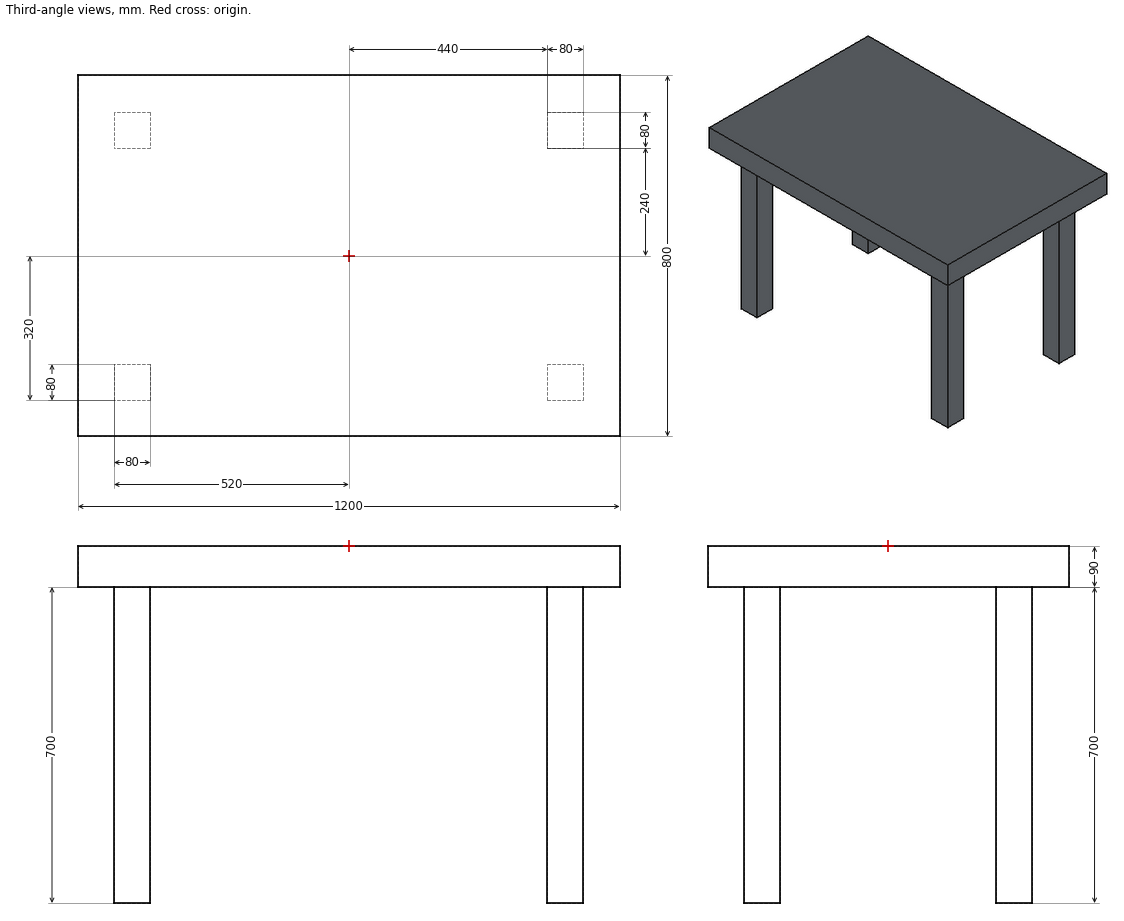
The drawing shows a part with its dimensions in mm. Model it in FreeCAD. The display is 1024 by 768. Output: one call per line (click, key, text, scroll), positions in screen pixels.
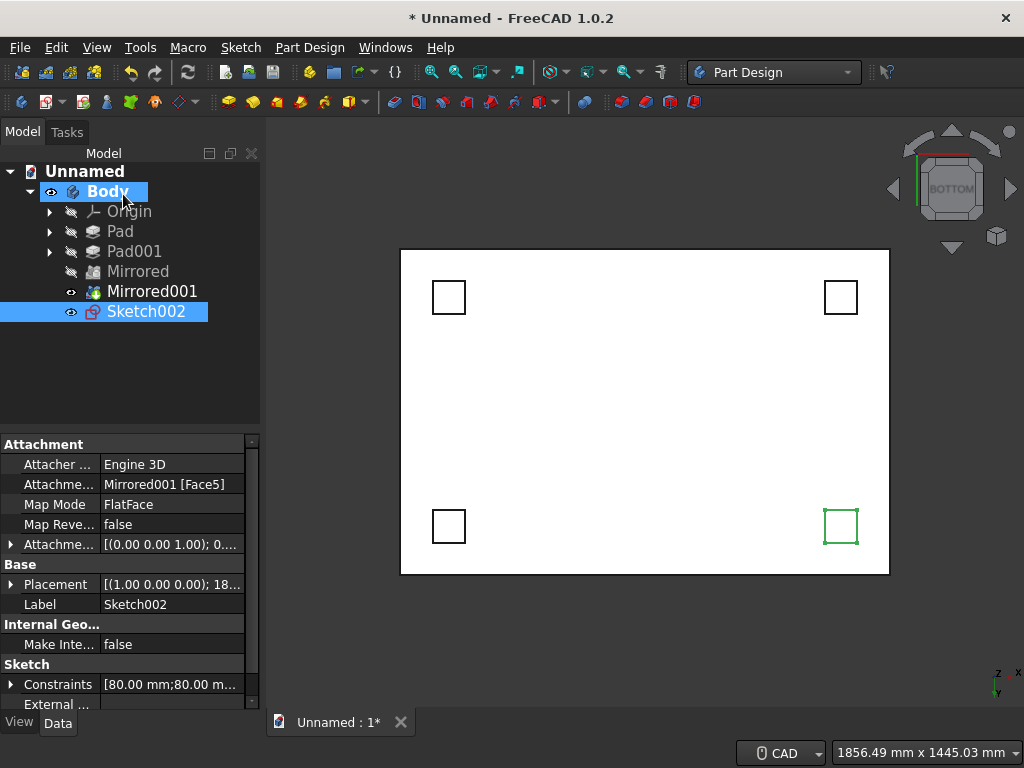
click(230, 102)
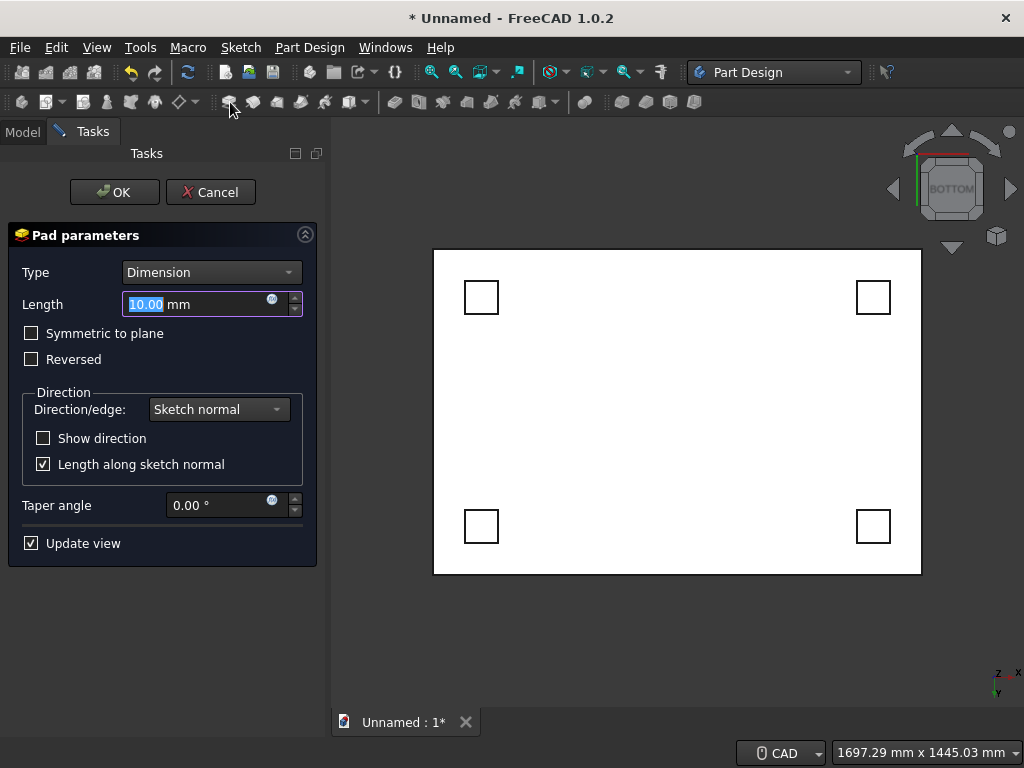
text(700)
key(Tab)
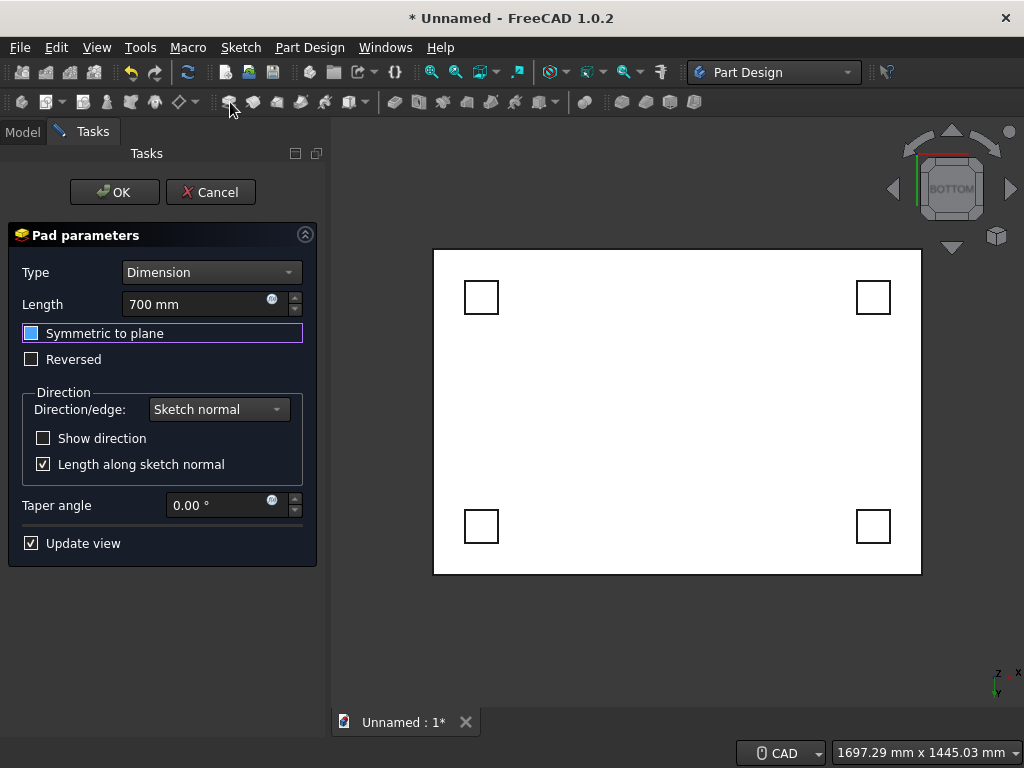
click(115, 192)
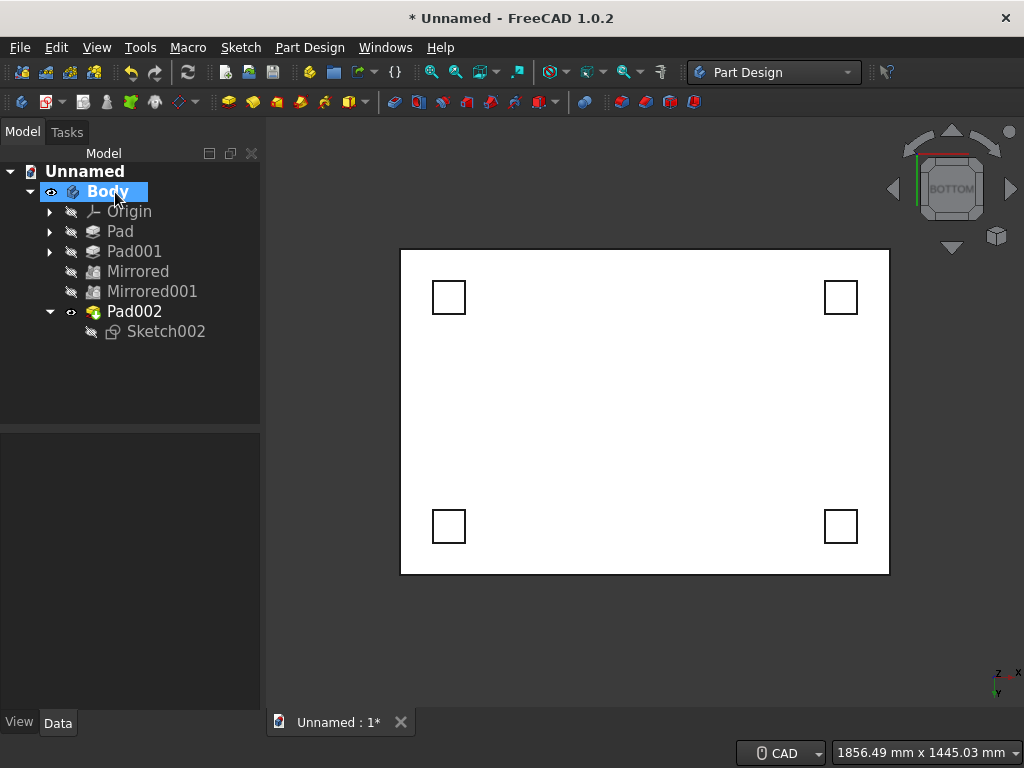
key(0)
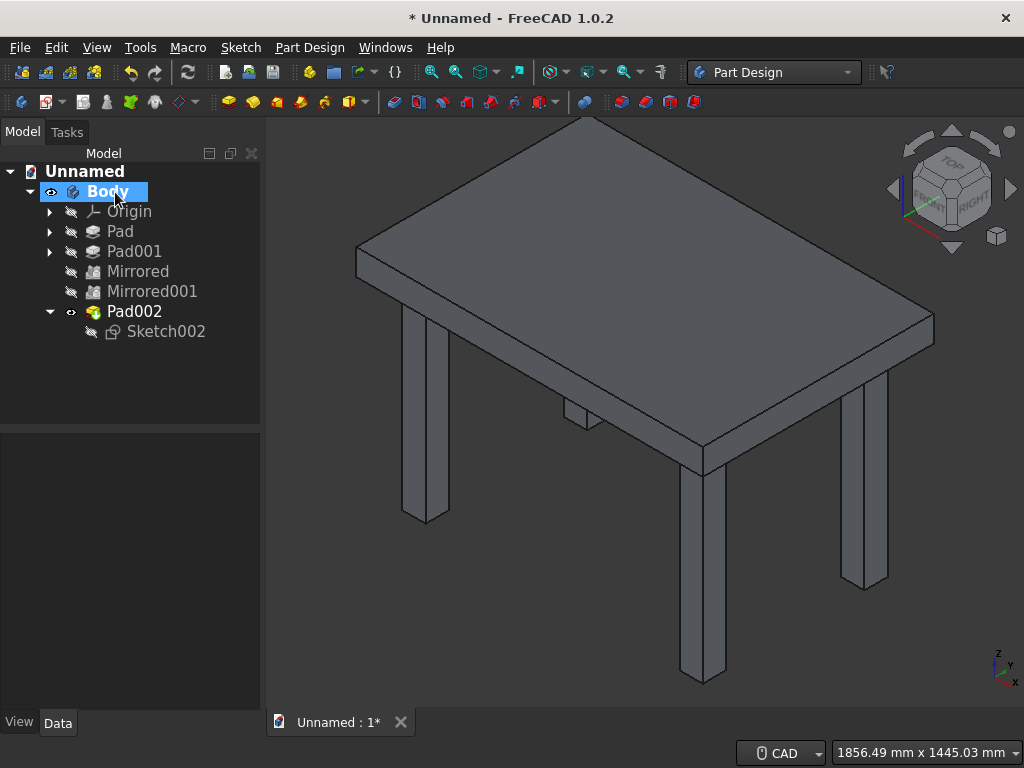
click(432, 72)